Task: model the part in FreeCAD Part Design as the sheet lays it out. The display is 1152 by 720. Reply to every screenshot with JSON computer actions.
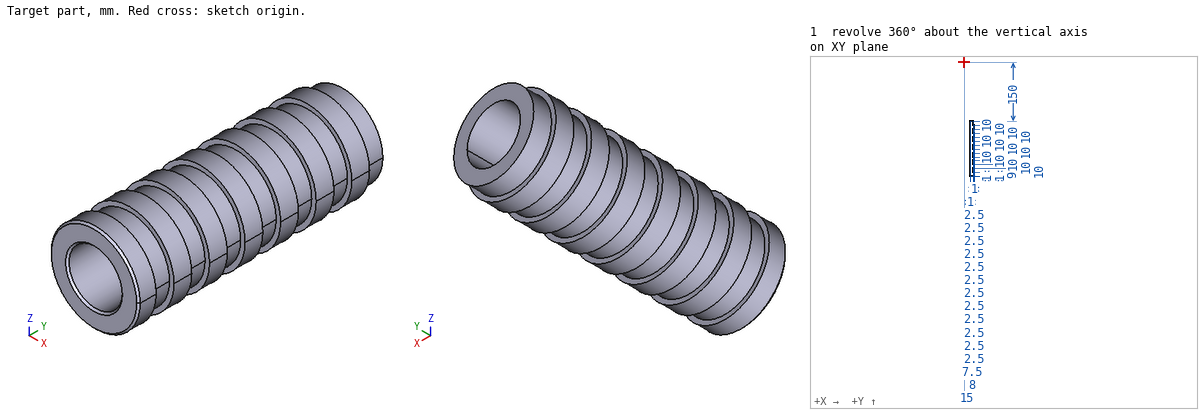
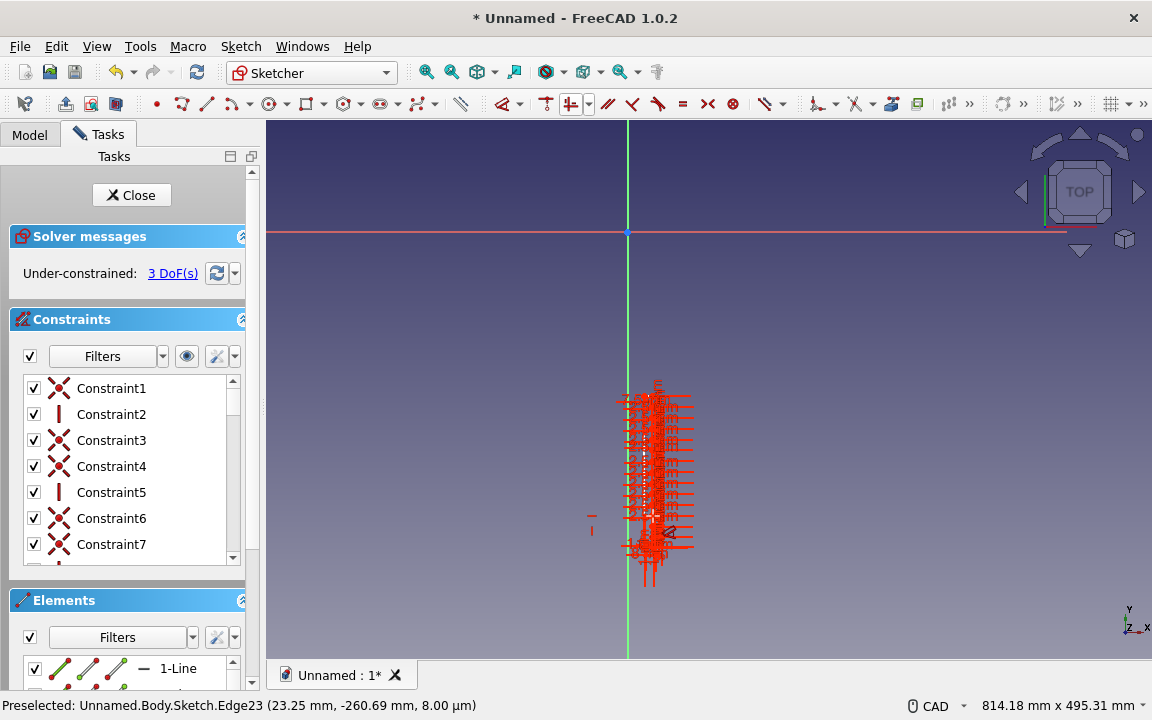
{"action": "scroll", "coordinate": [654, 527], "scroll_direction": "up", "scroll_amount": 14}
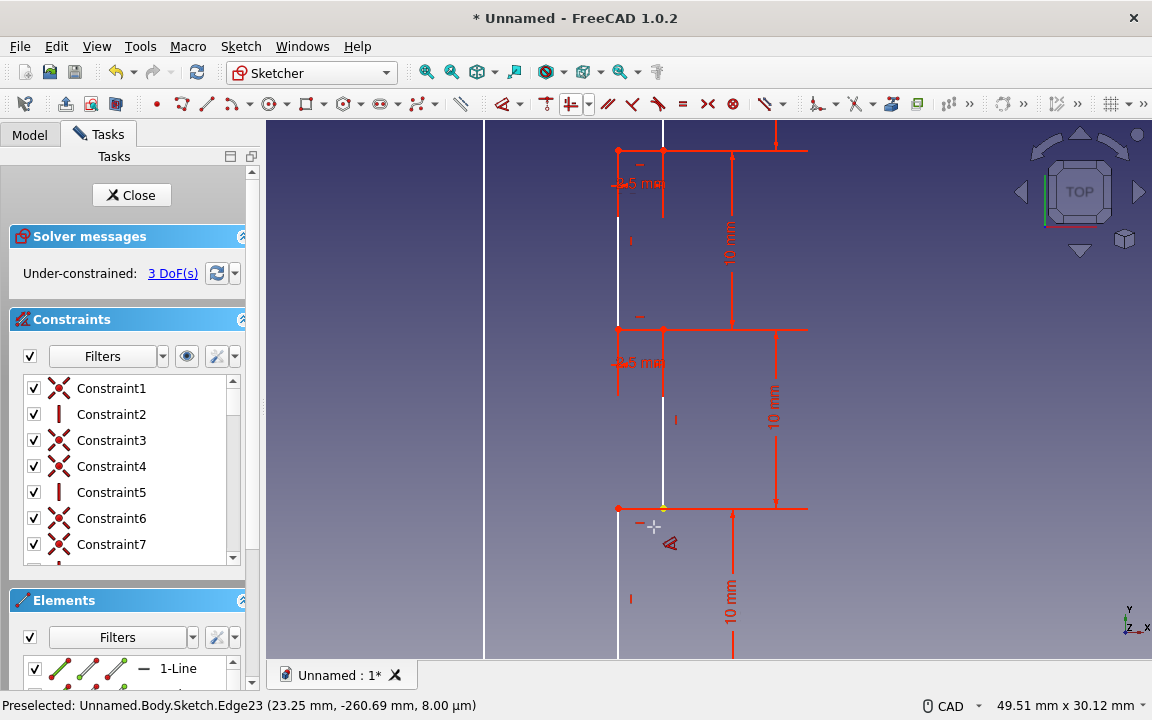
{"action": "left_click", "coordinate": [650, 509]}
{"action": "left_click", "coordinate": [641, 543]}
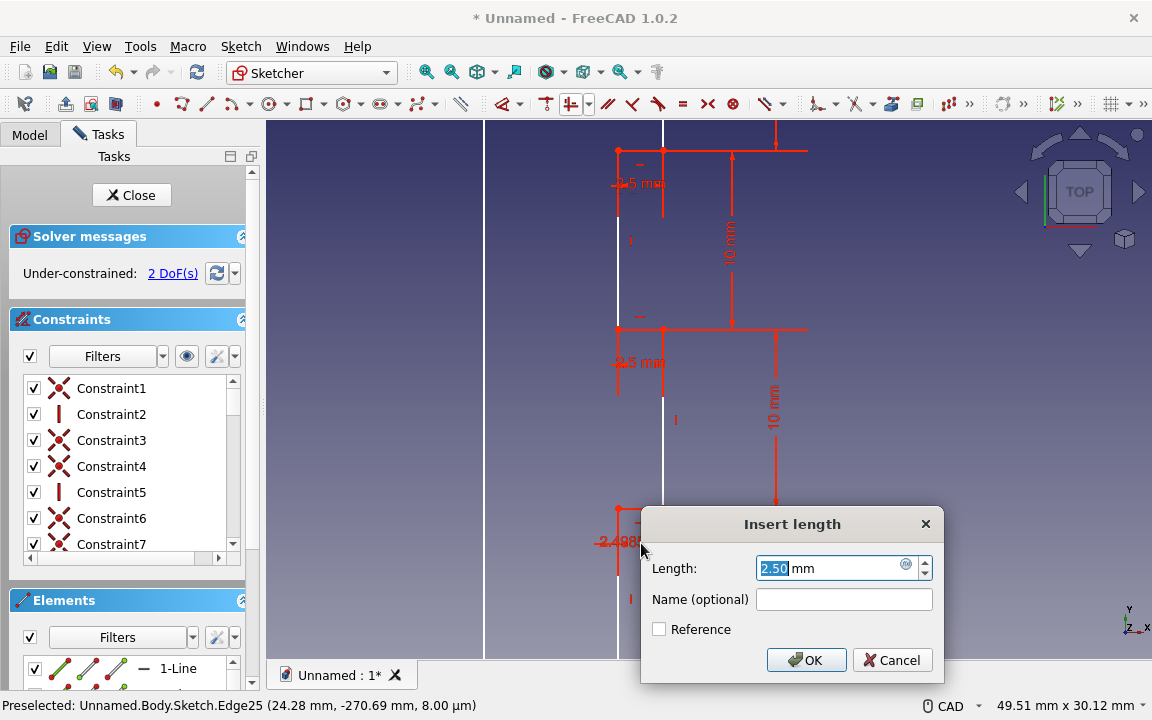
{"action": "type", "text": "2.5"}
{"action": "key", "text": "Return"}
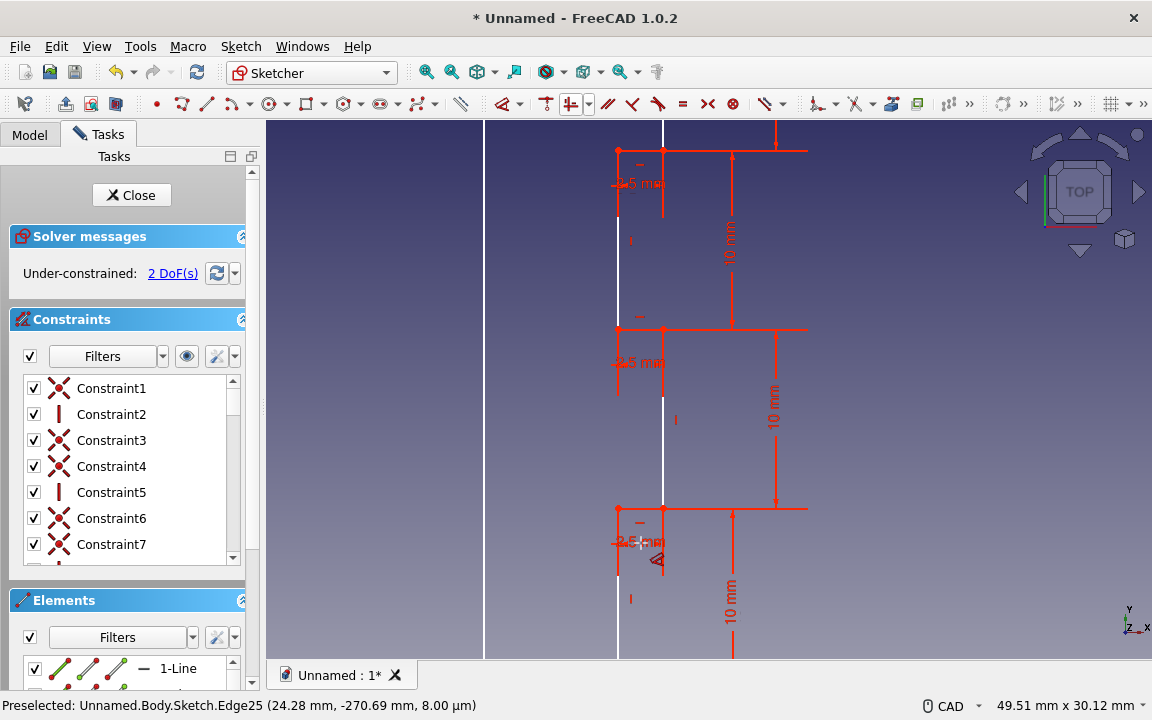
{"action": "scroll", "coordinate": [654, 527], "scroll_direction": "down", "scroll_amount": 14}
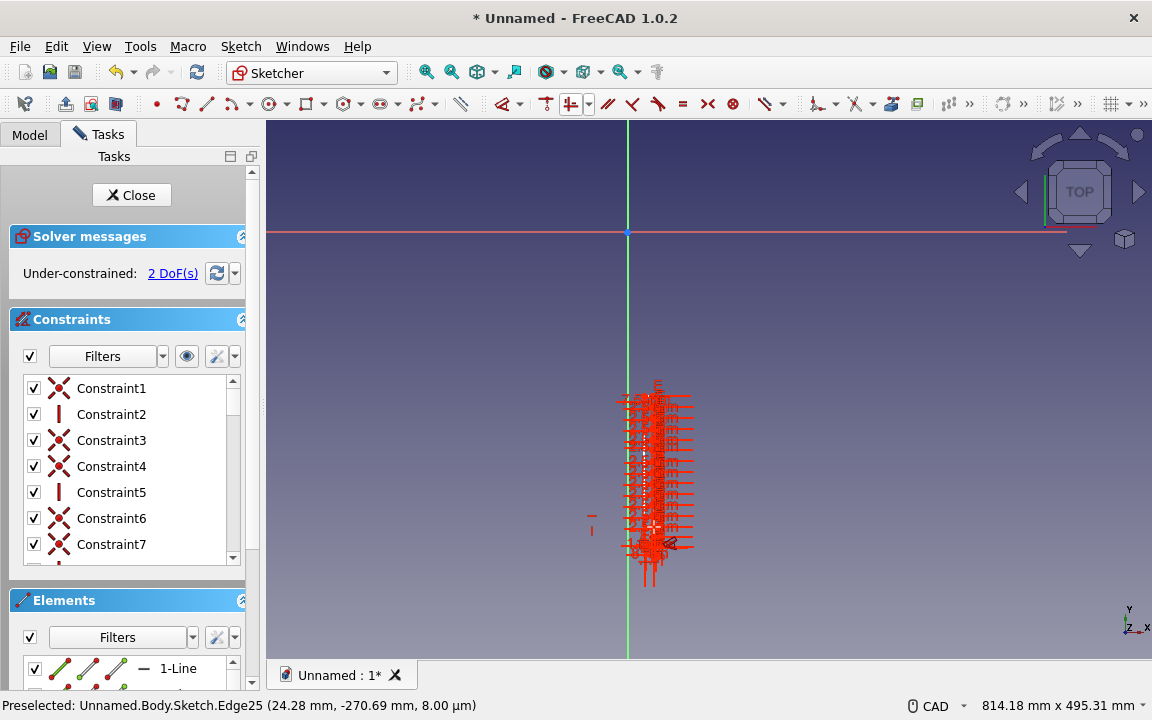
{"action": "scroll", "coordinate": [644, 396], "scroll_direction": "up", "scroll_amount": 5}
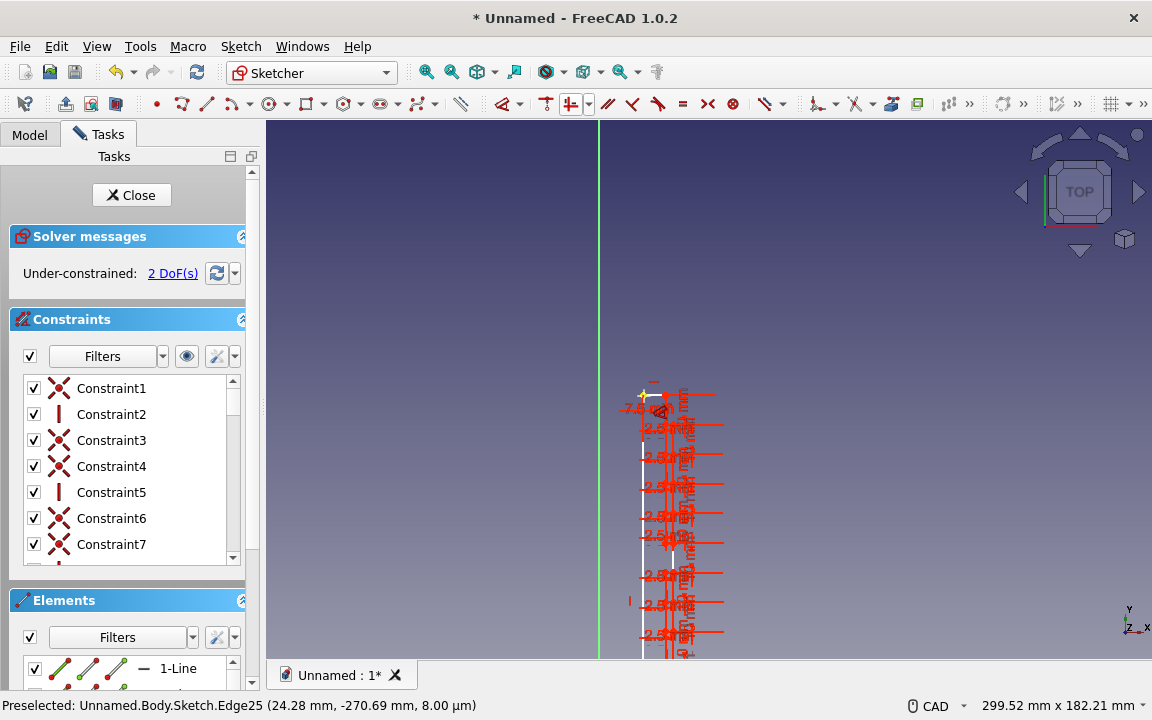
{"action": "left_click", "coordinate": [643, 395]}
{"action": "left_click", "coordinate": [621, 429]}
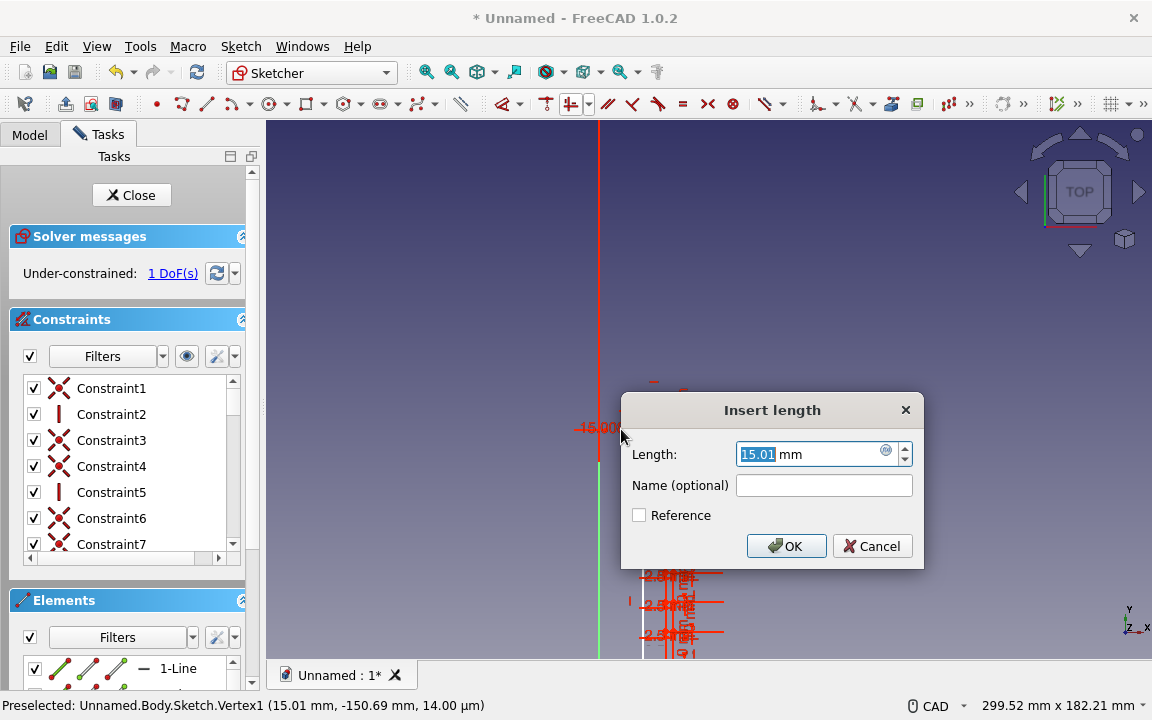
{"action": "type", "text": "15"}
{"action": "key", "text": "Return"}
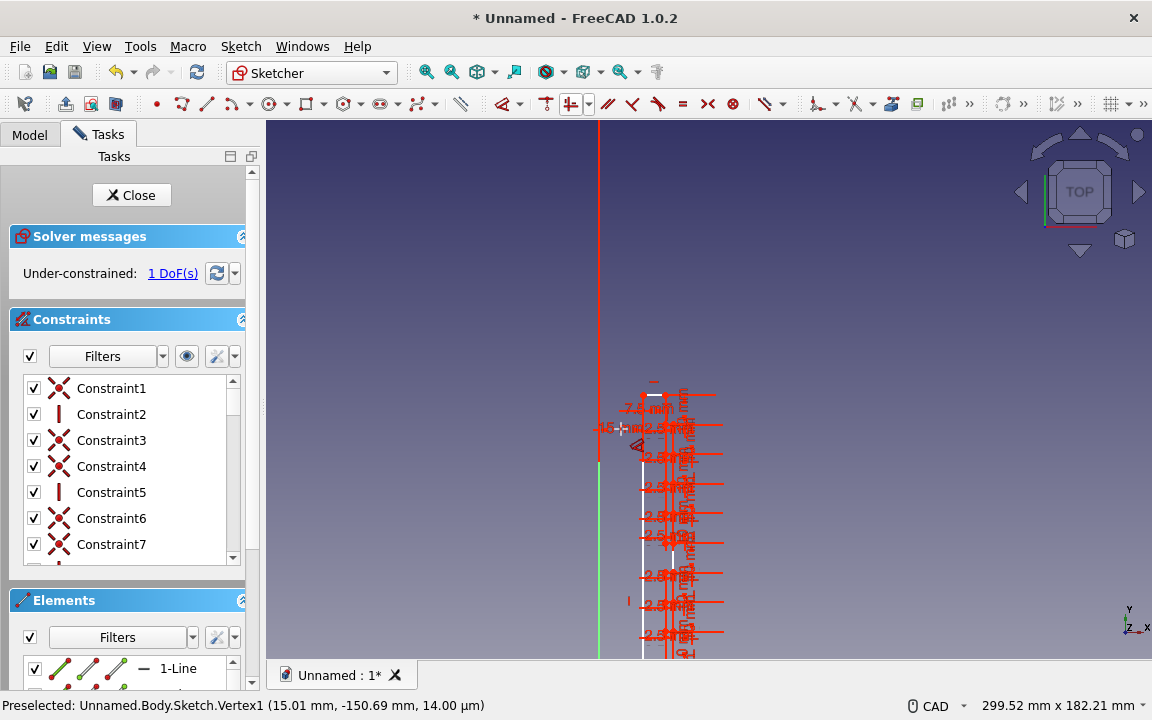
{"action": "left_click", "coordinate": [643, 395]}
{"action": "left_click", "coordinate": [565, 272]}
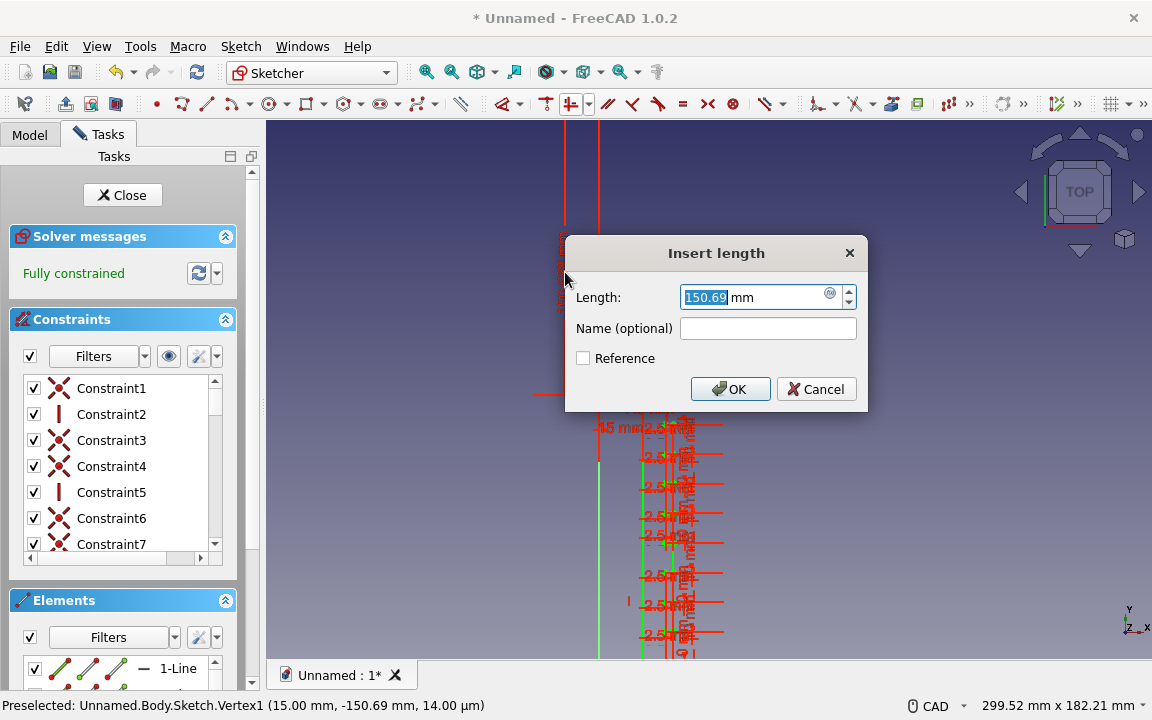
{"action": "type", "text": "150"}
{"action": "key", "text": "Return"}
{"action": "key", "text": "Escape"}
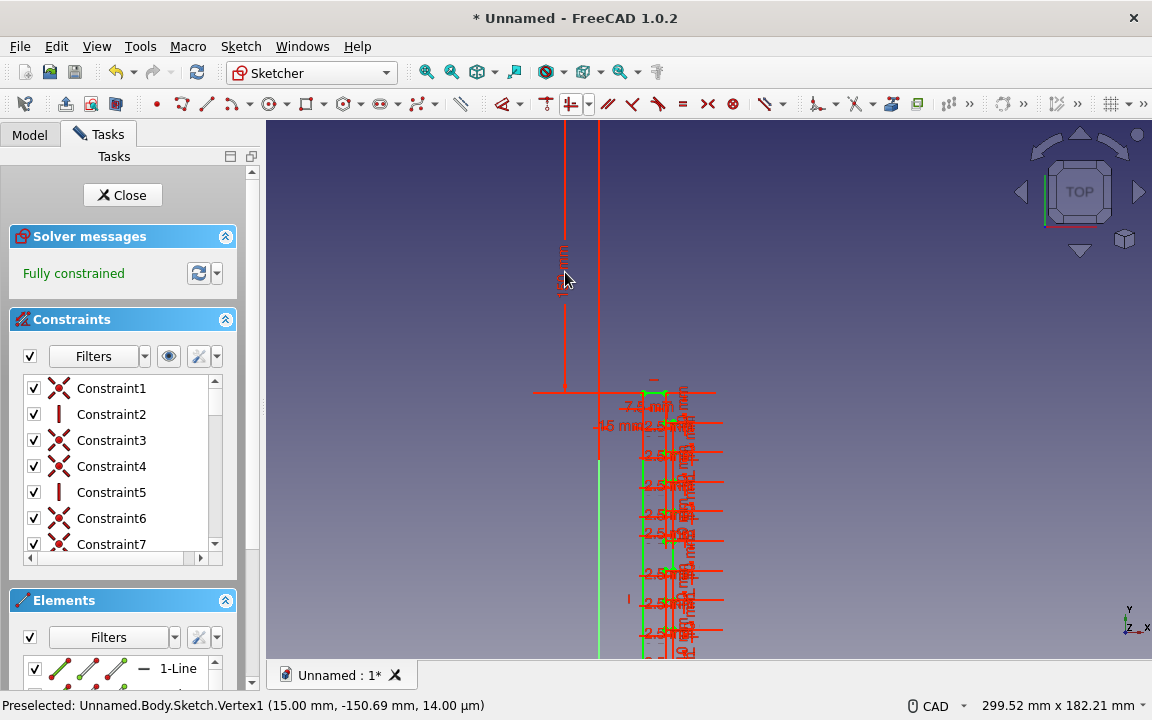
{"action": "left_click", "coordinate": [123, 195]}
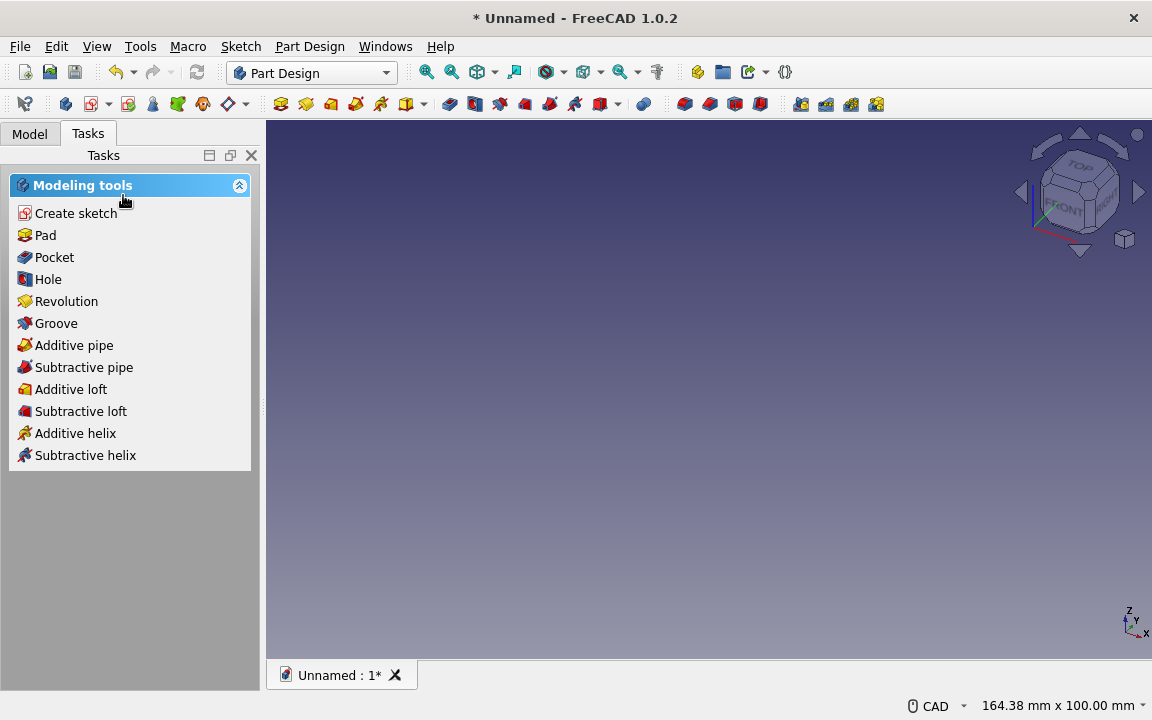
{"action": "left_click", "coordinate": [306, 104]}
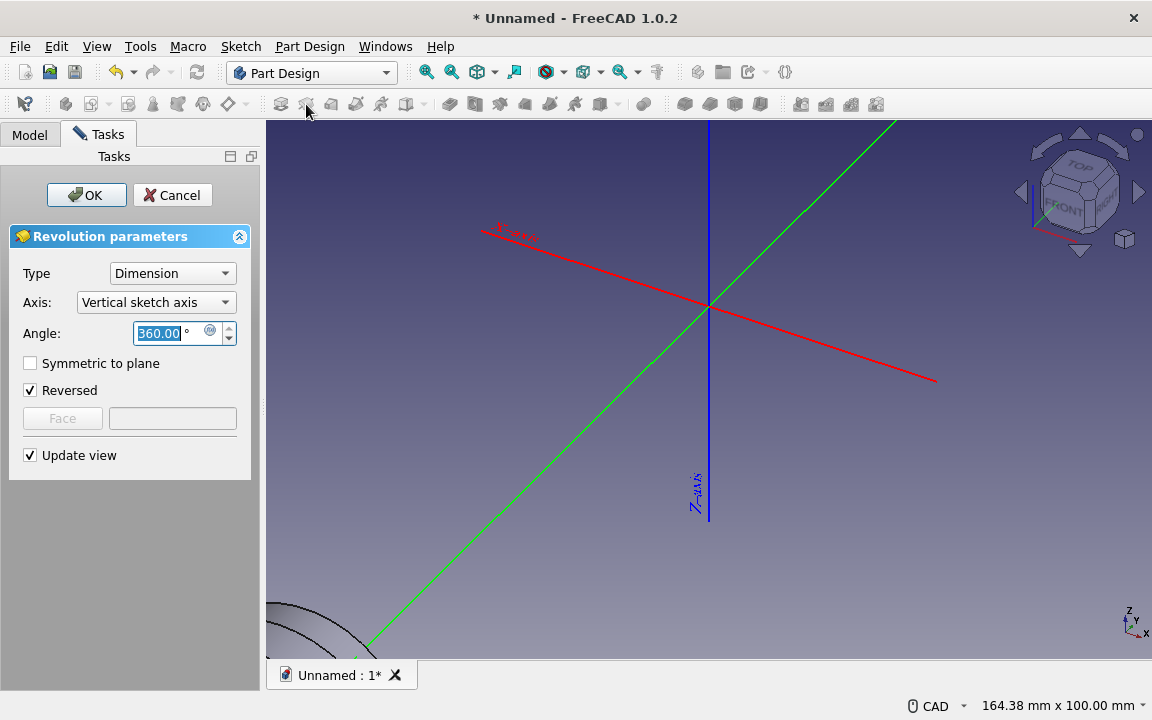
{"action": "left_click", "coordinate": [87, 195]}